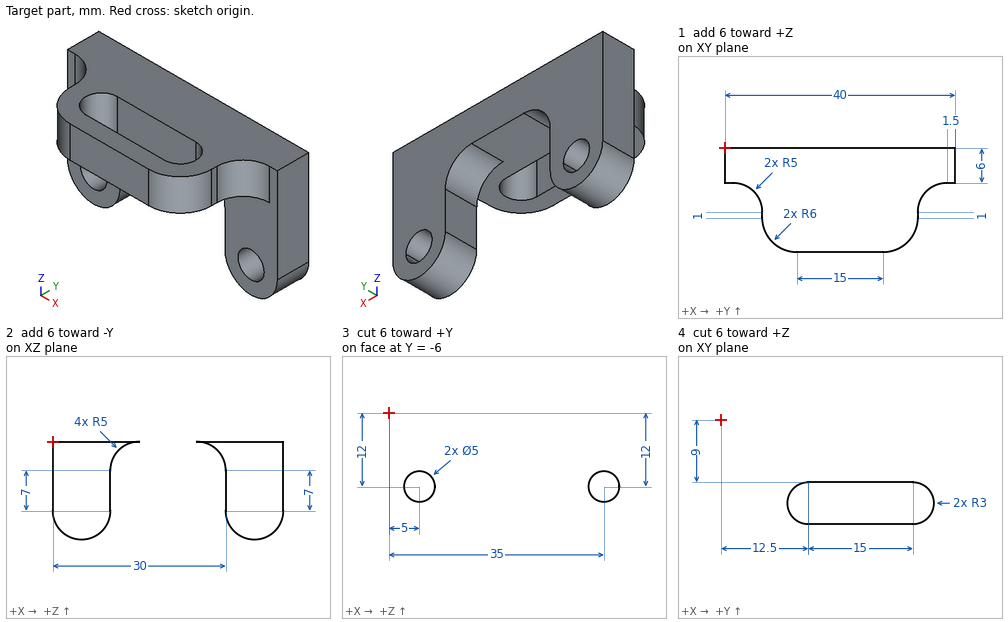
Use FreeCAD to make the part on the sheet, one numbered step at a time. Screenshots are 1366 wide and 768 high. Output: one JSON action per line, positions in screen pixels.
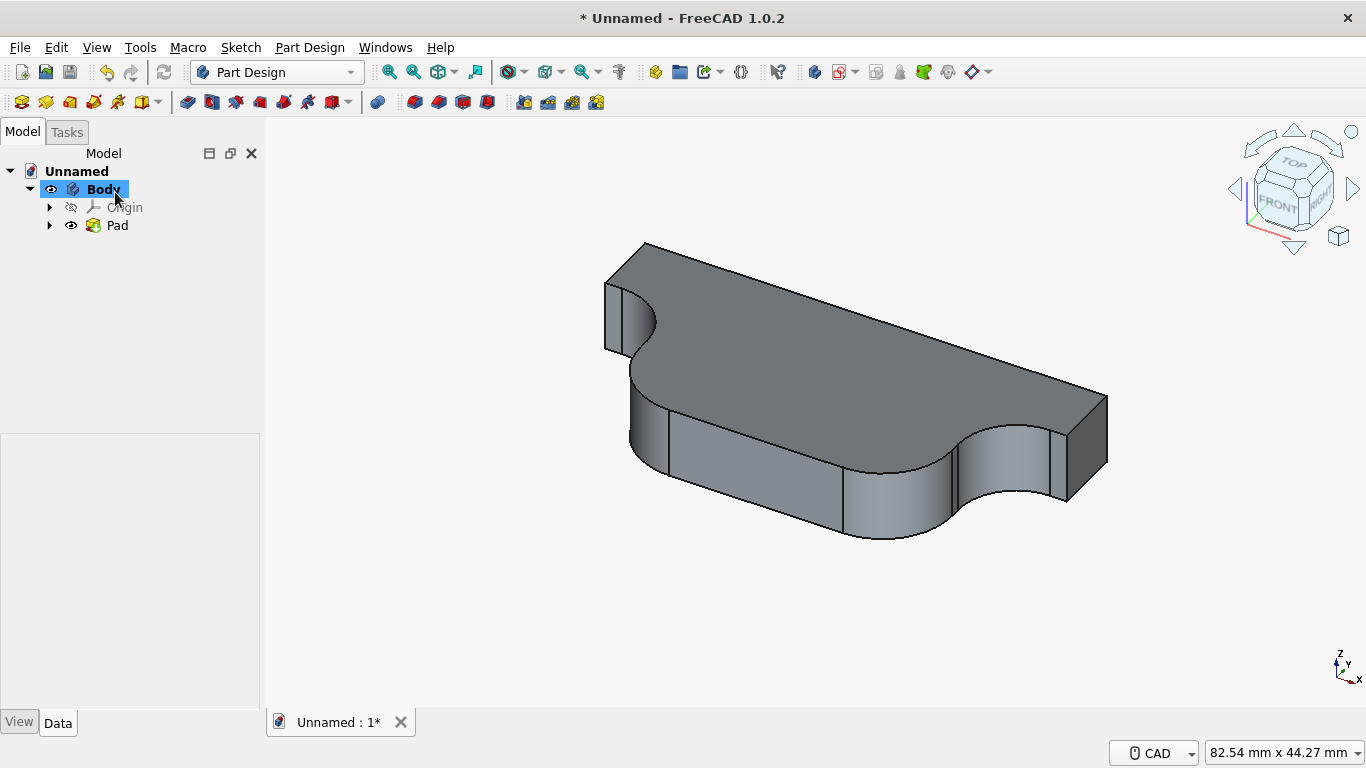
{"action": "left_click", "coordinate": [840, 72]}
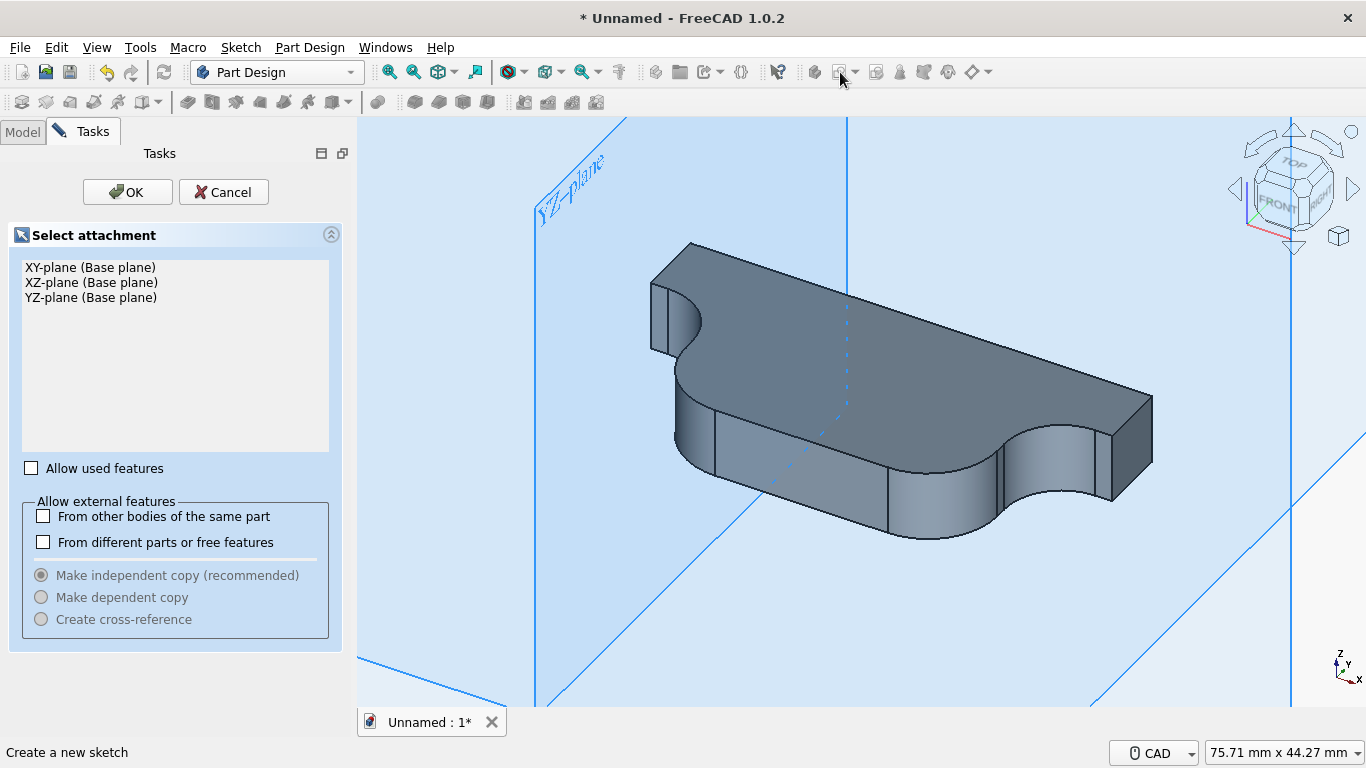
{"action": "left_click", "coordinate": [82, 282]}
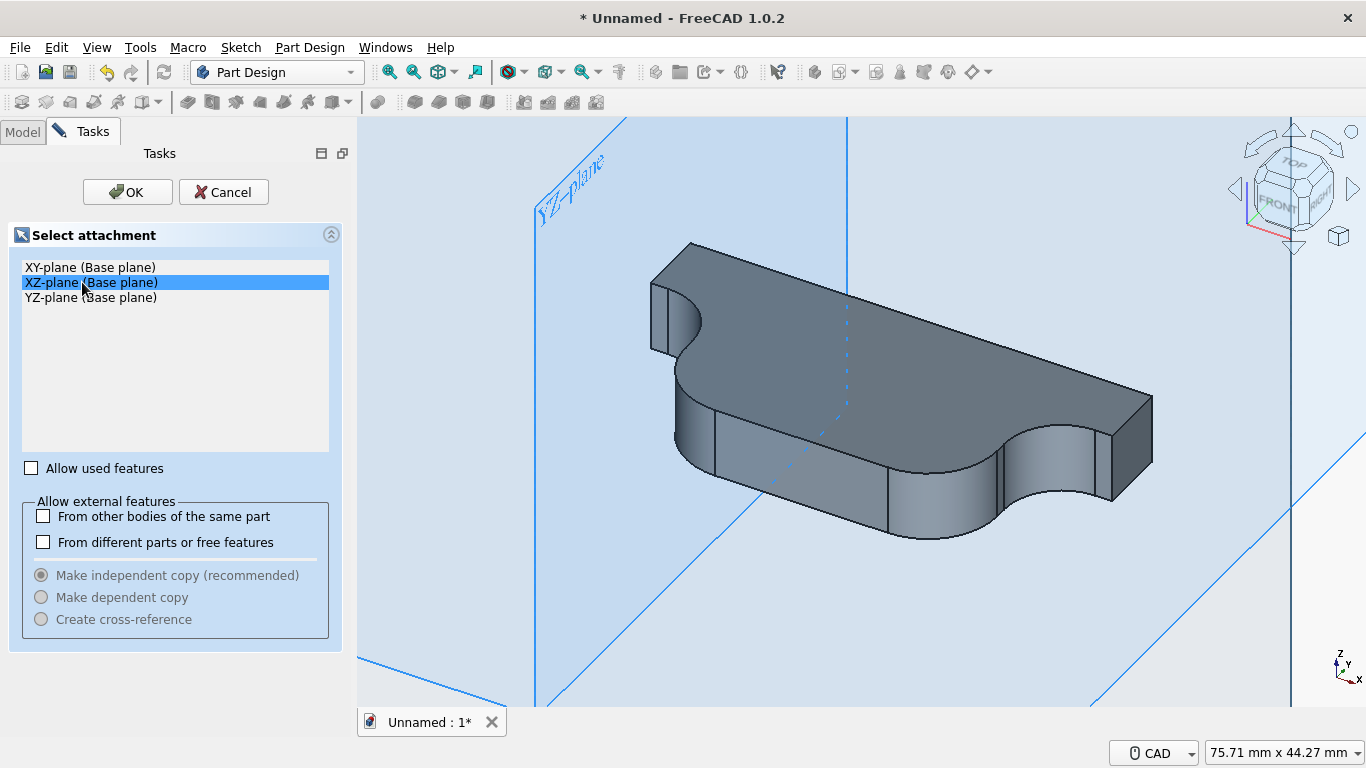
{"action": "left_click", "coordinate": [128, 192]}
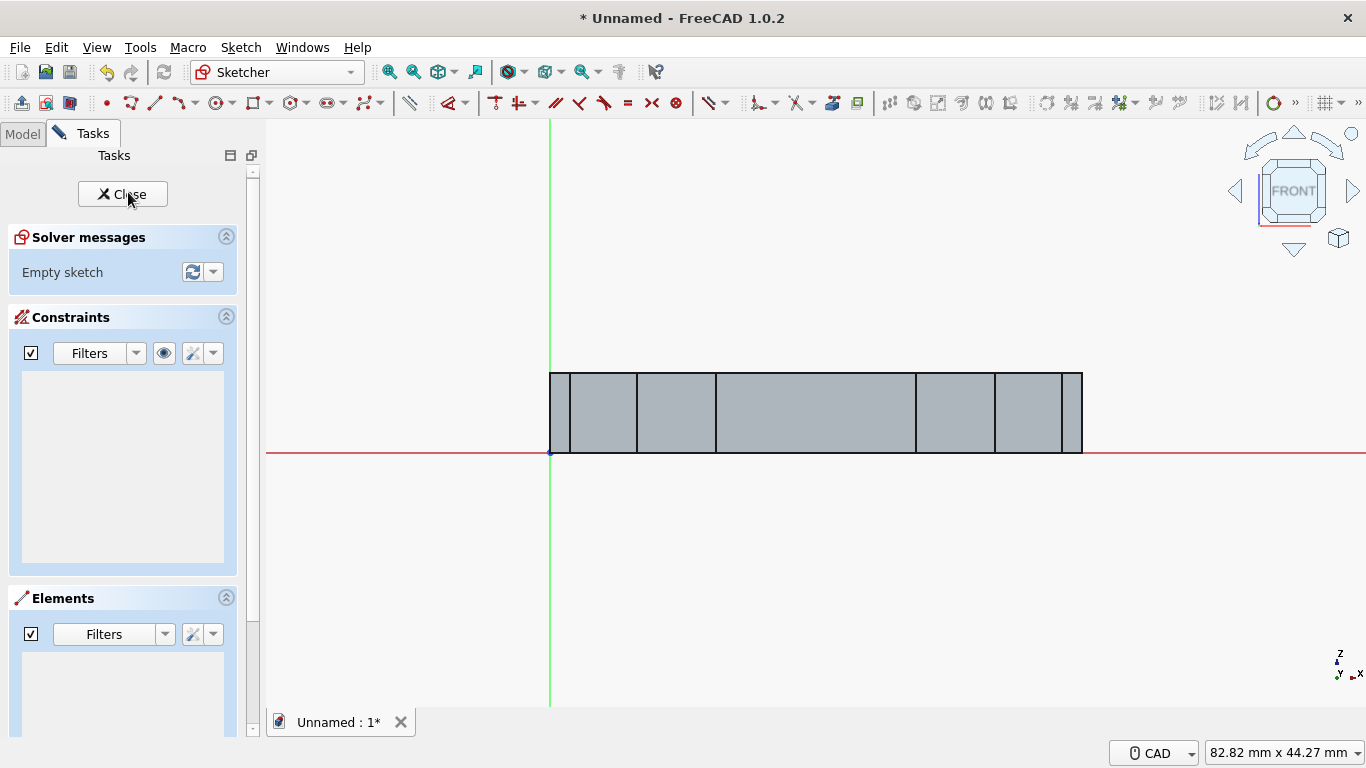
{"action": "key", "text": "q s"}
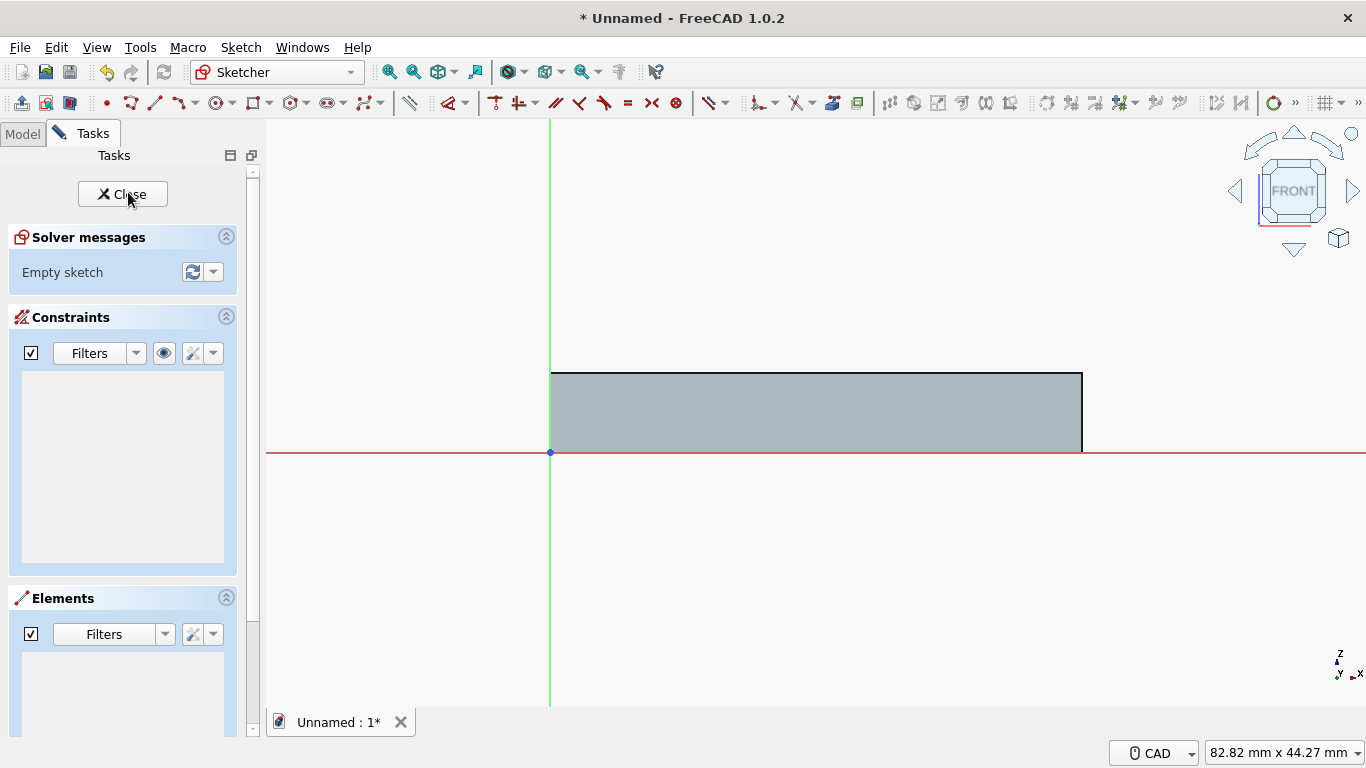
{"action": "scroll", "coordinate": [438, 147], "scroll_direction": "down", "scroll_amount": 1}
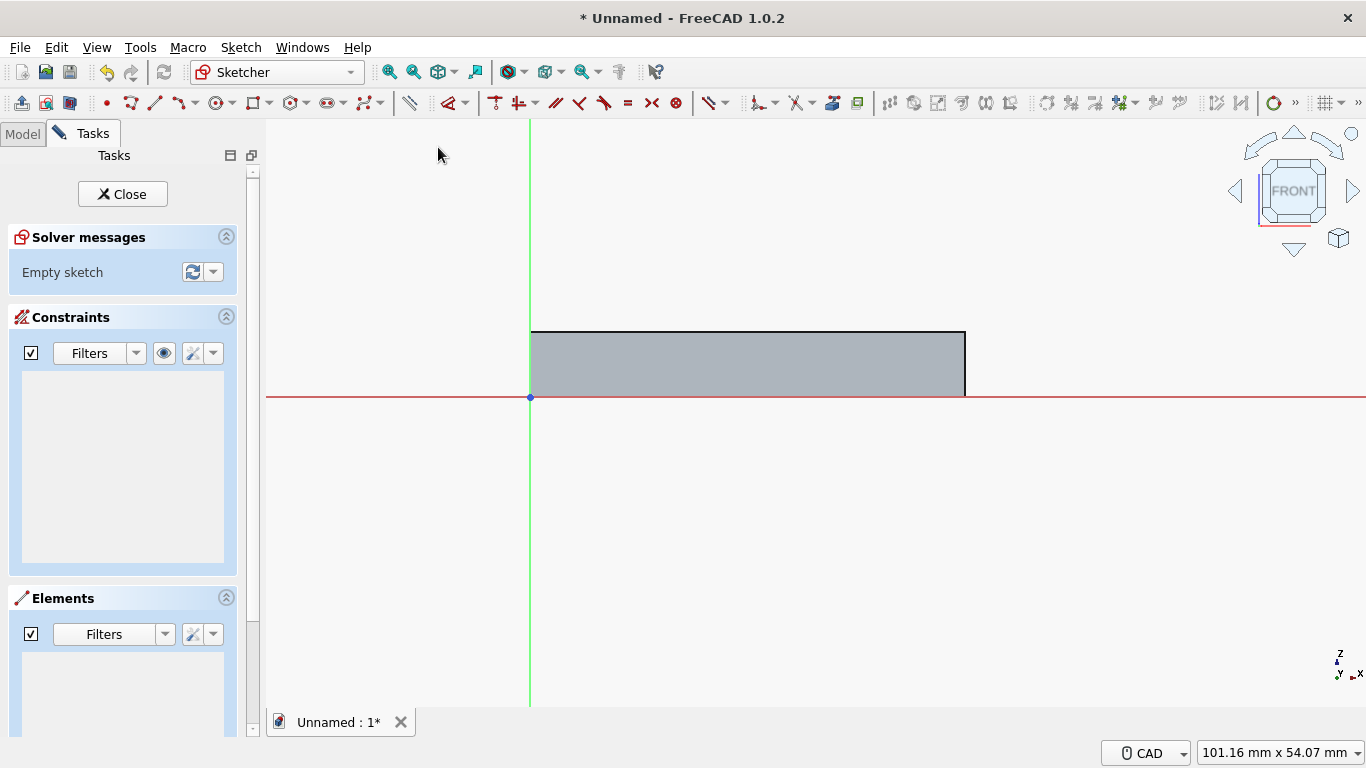
{"action": "scroll", "coordinate": [748, 646], "scroll_direction": "up", "scroll_amount": 2}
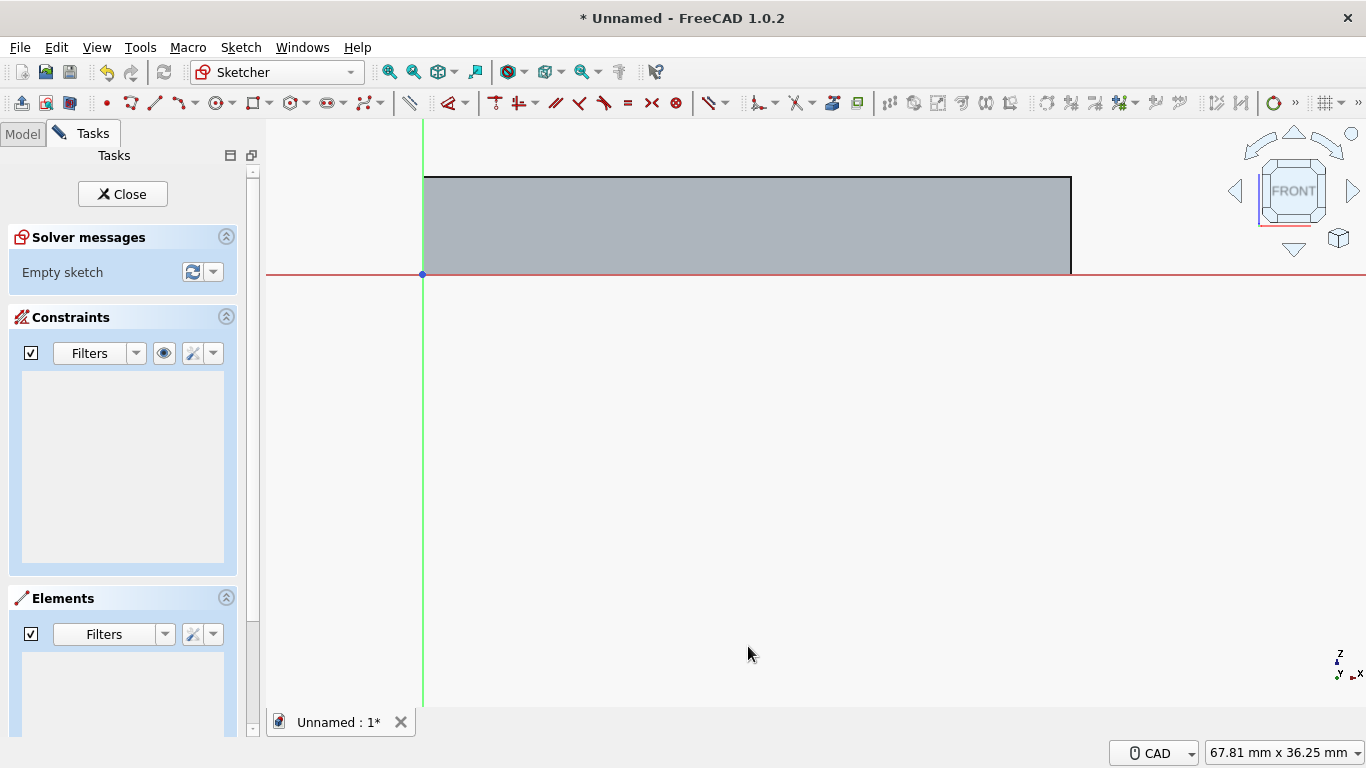
{"action": "key", "text": "g m"}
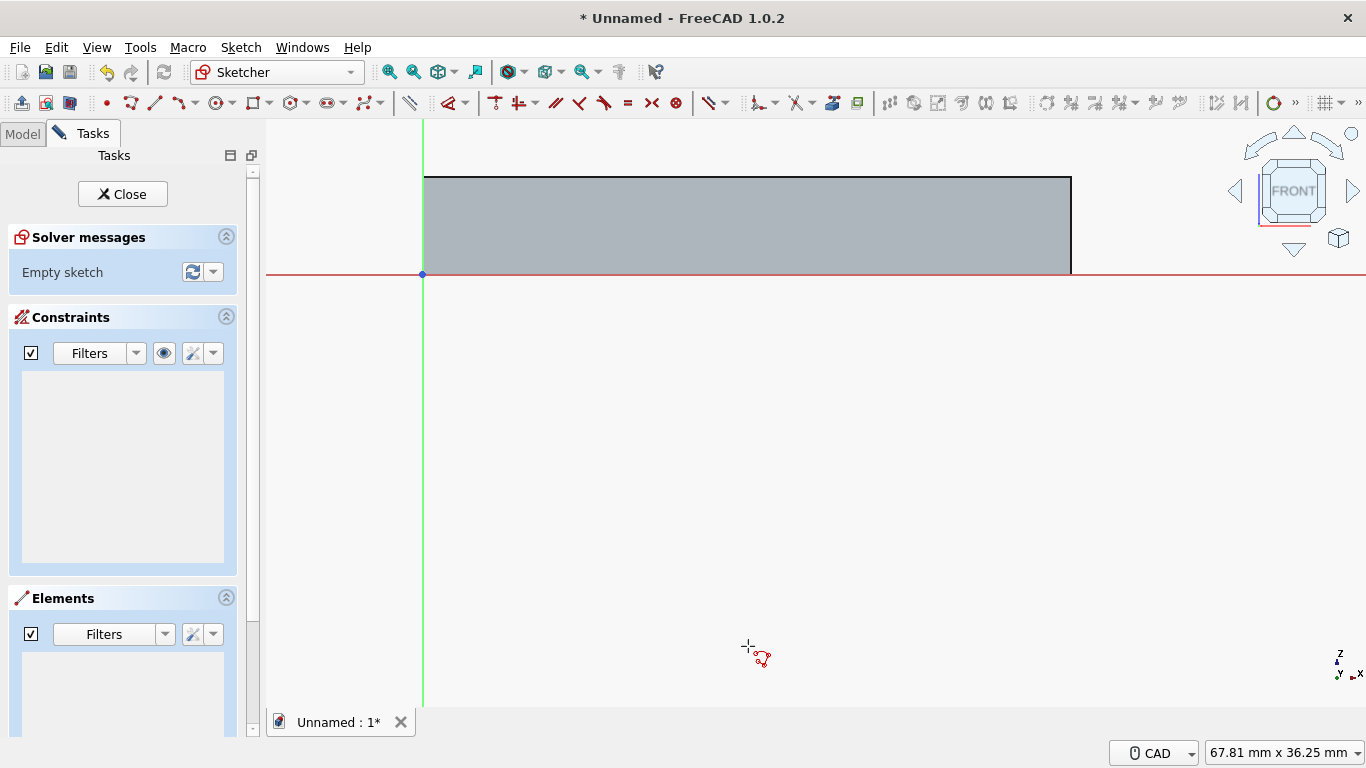
{"action": "left_click", "coordinate": [423, 469]}
{"action": "left_click", "coordinate": [423, 275]}
{"action": "left_click", "coordinate": [666, 284]}
{"action": "right_click", "coordinate": [666, 284]}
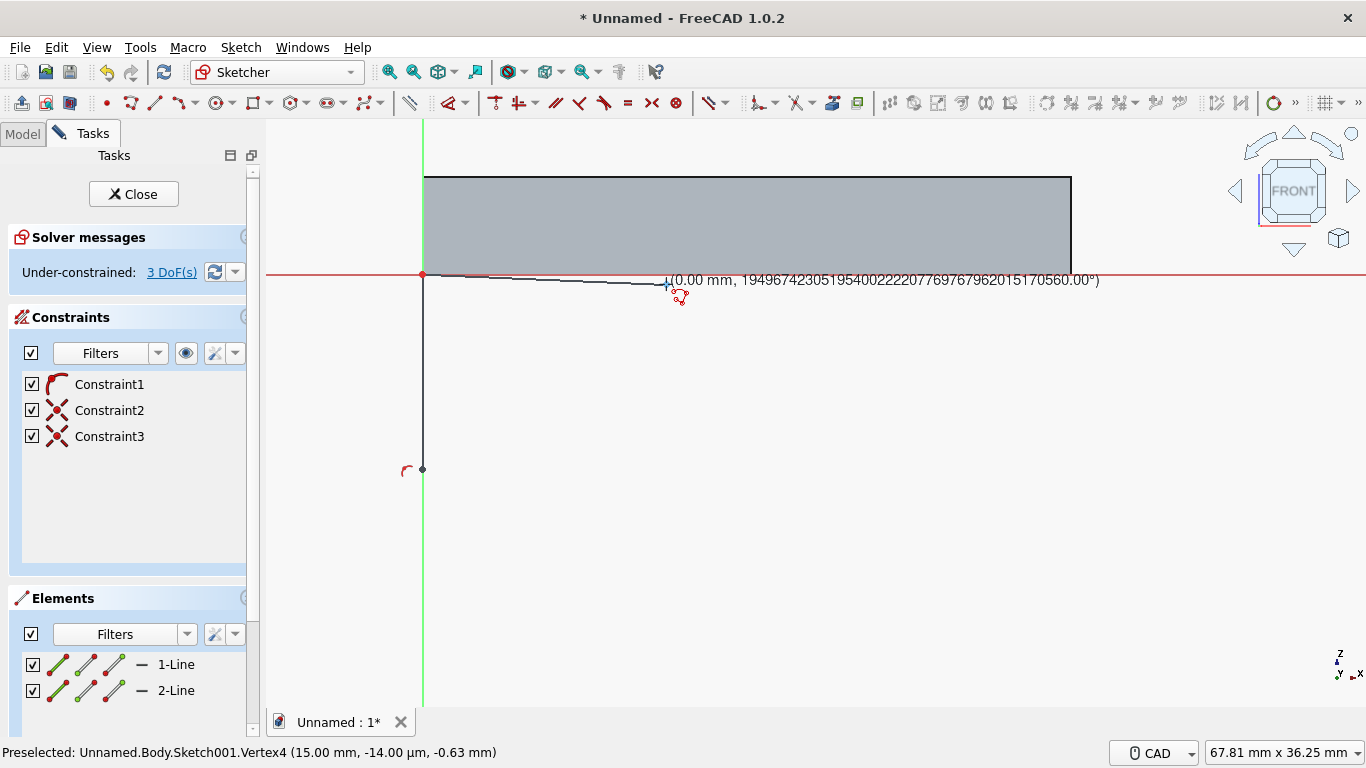
{"action": "left_click", "coordinate": [156, 104]}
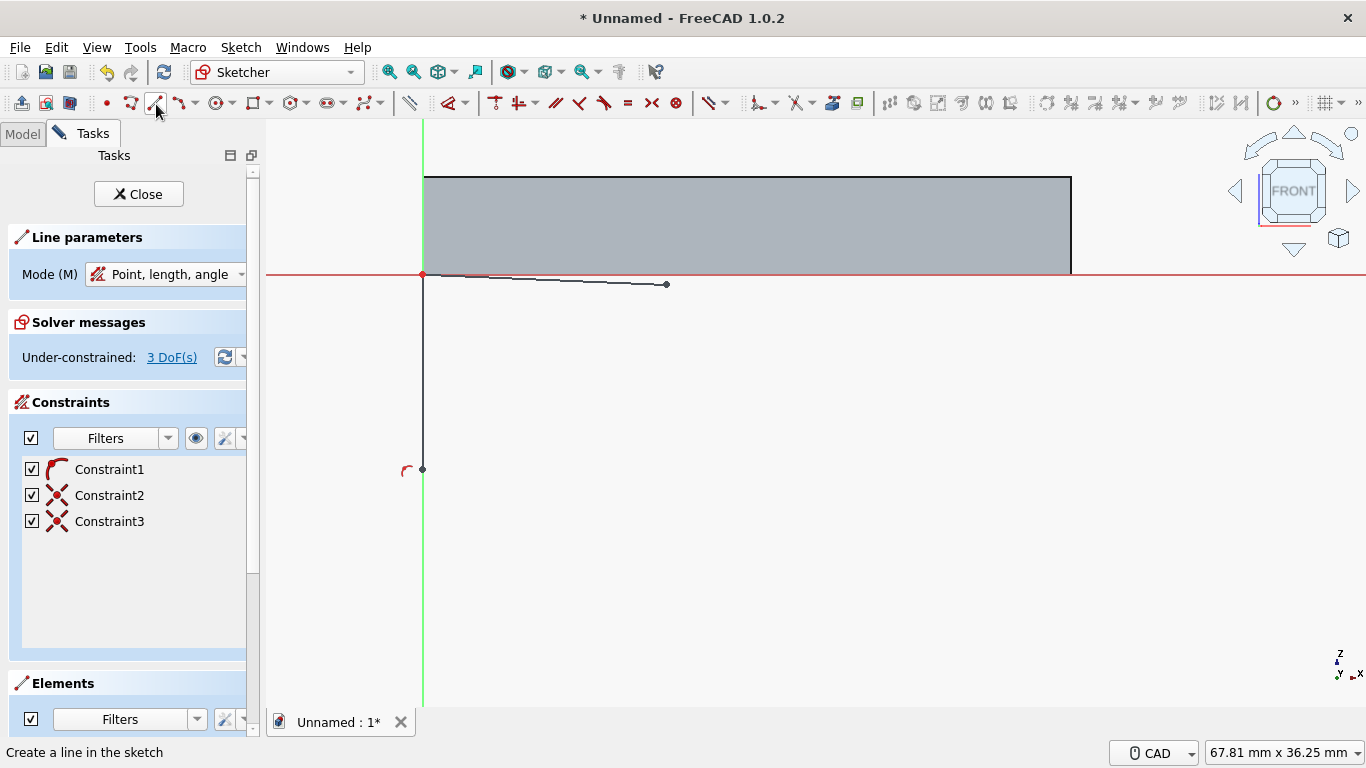
{"action": "left_click", "coordinate": [585, 356]}
{"action": "left_click", "coordinate": [585, 469]}